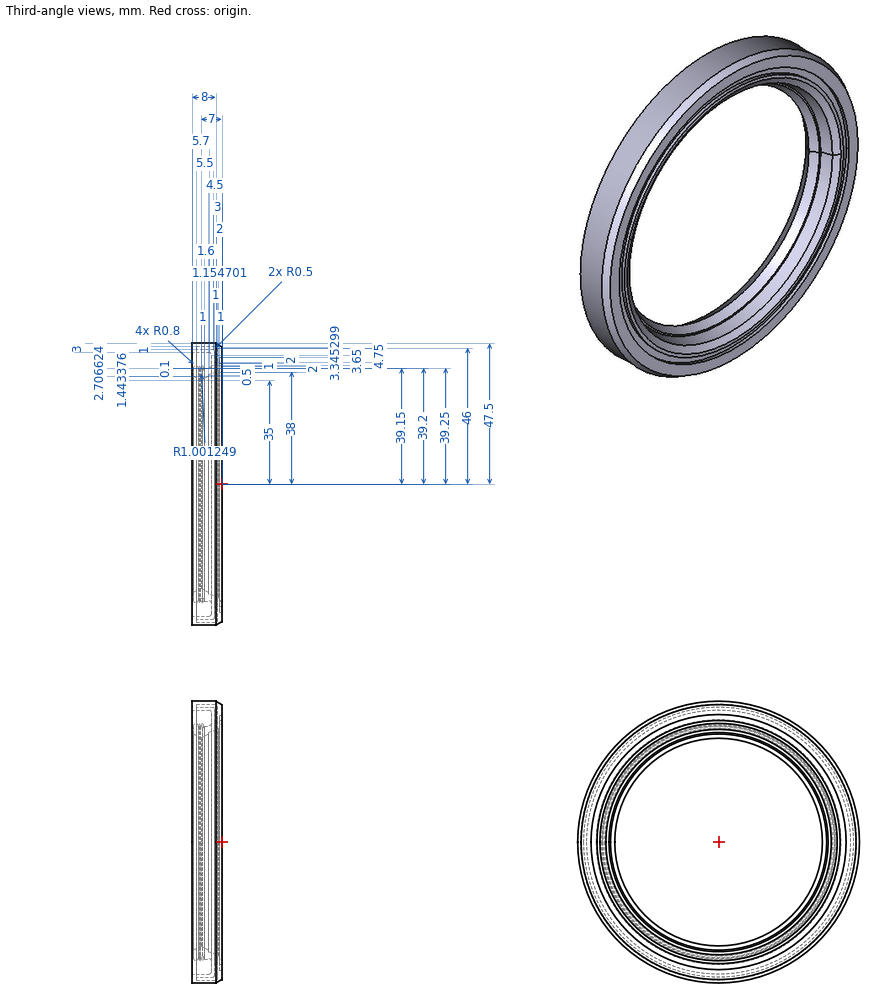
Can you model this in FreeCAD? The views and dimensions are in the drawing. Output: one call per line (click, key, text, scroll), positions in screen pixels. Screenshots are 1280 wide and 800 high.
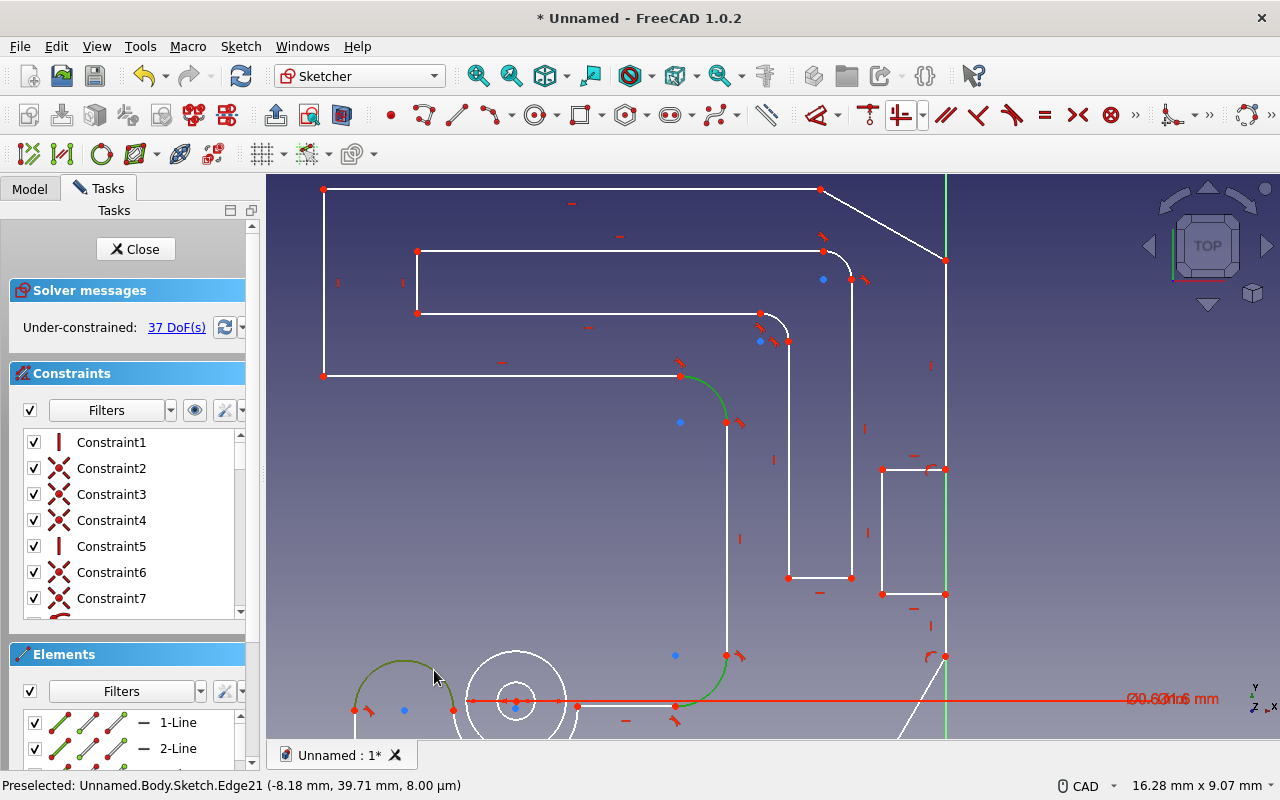
click(1045, 116)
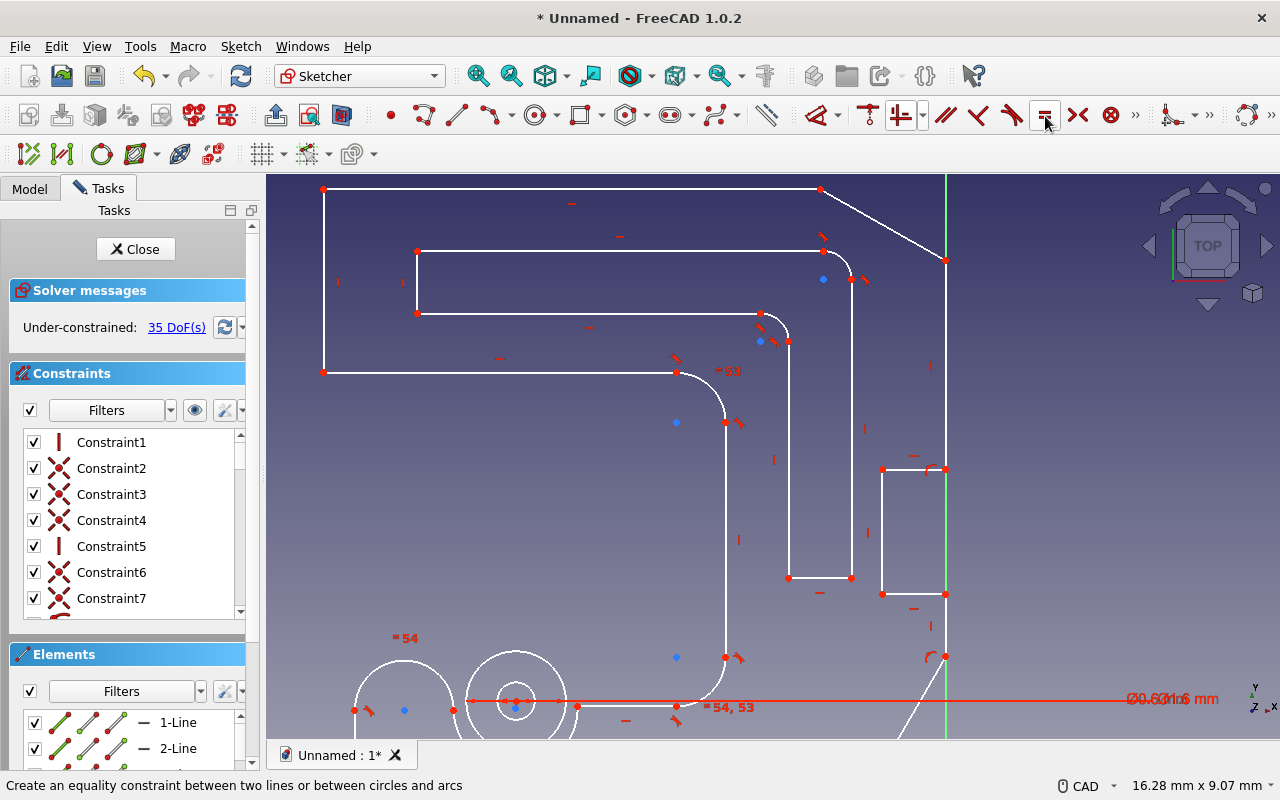
click(848, 266)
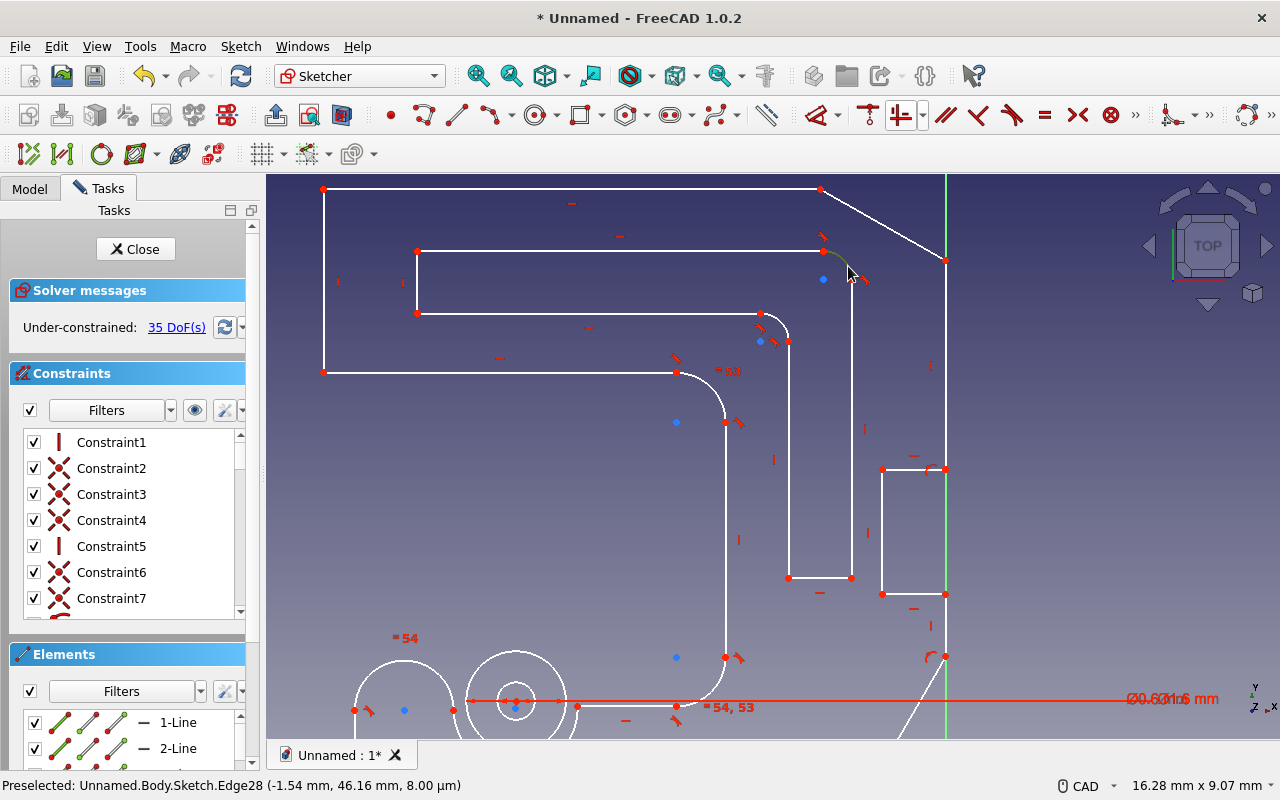
click(786, 329)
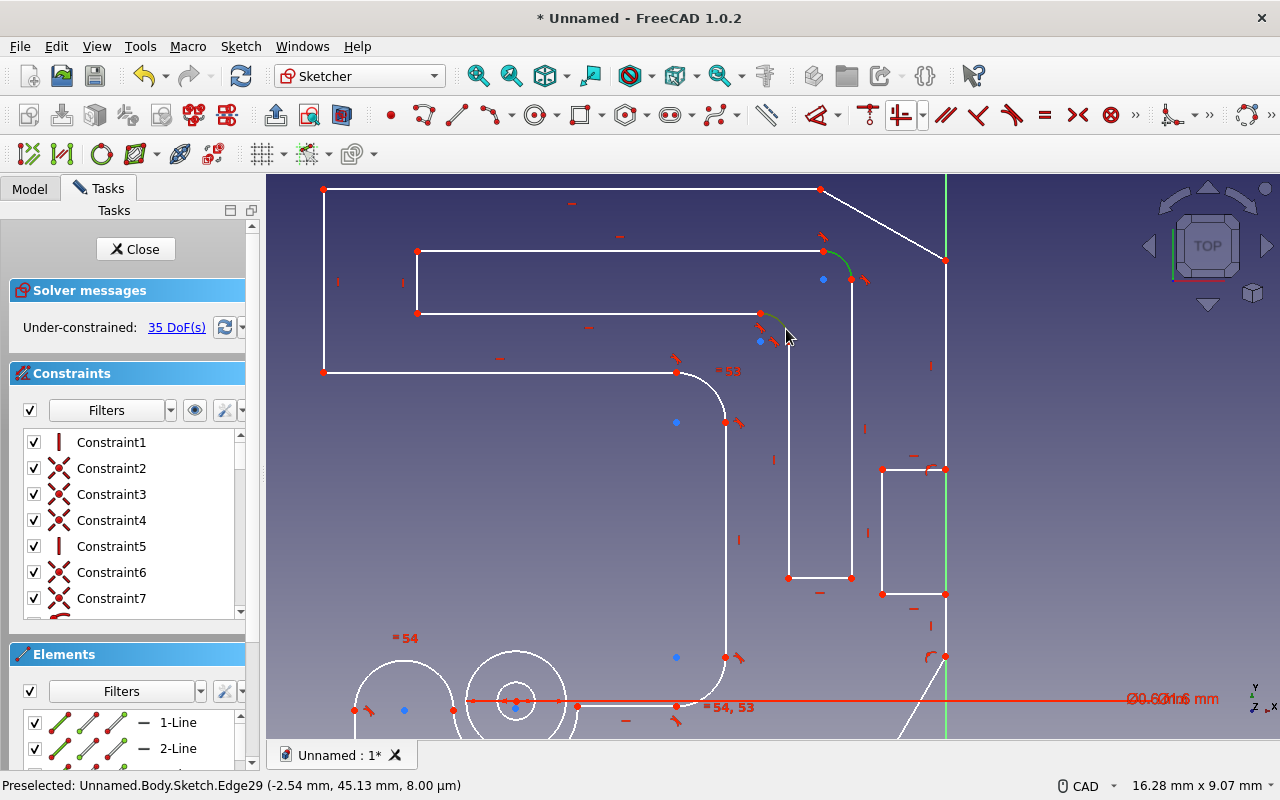
key(e)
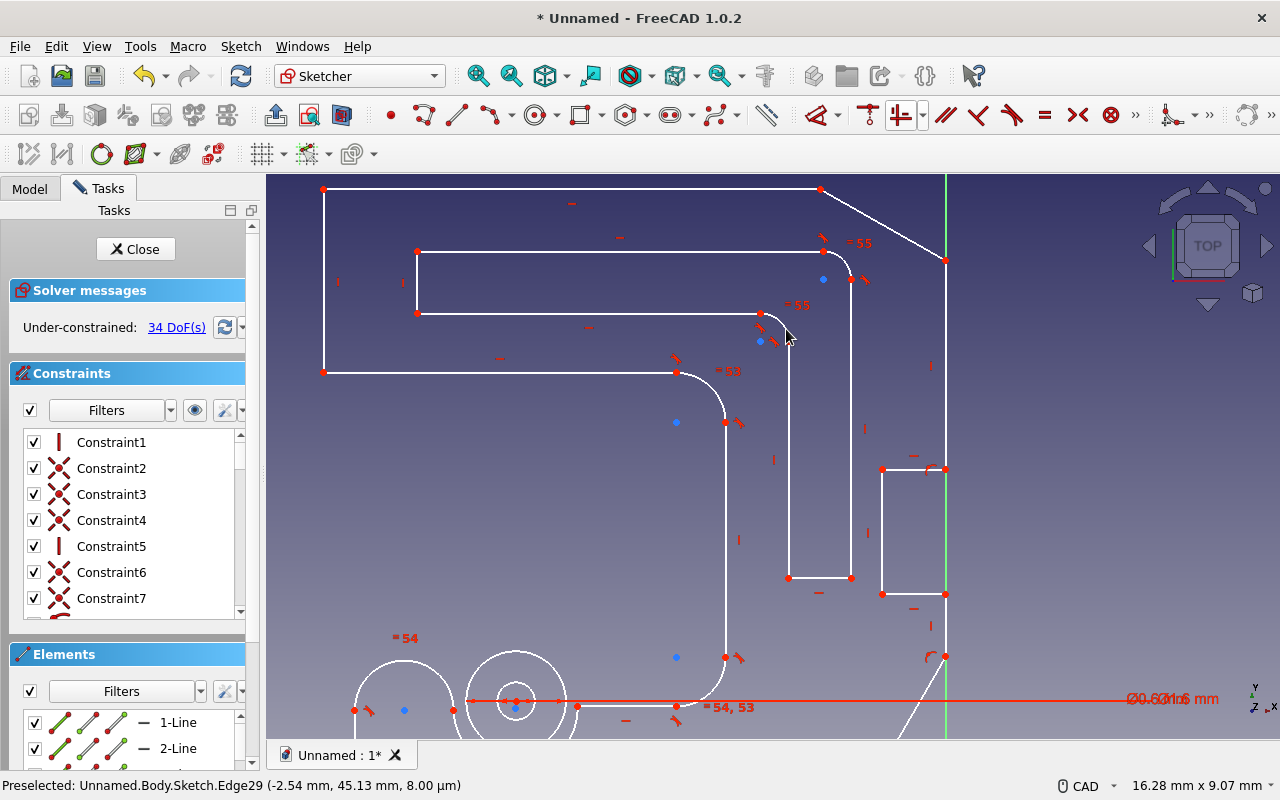
click(816, 116)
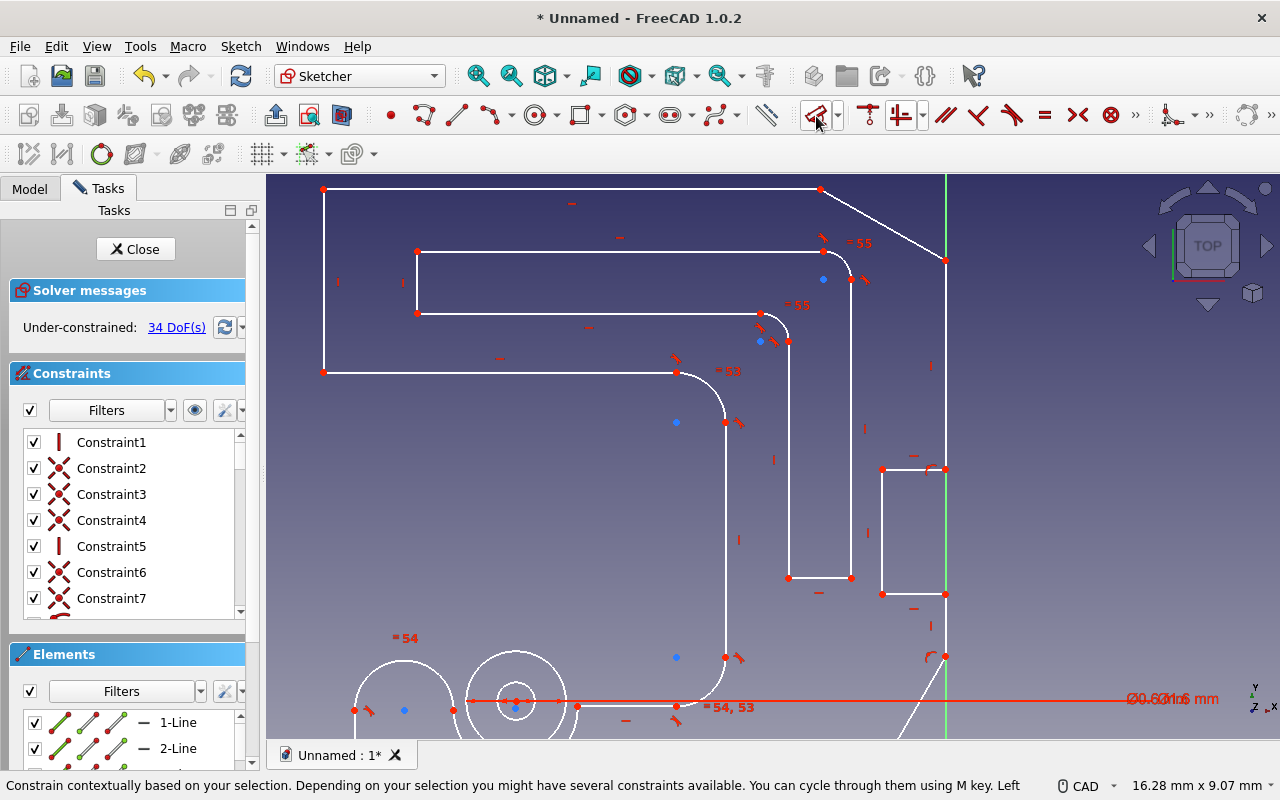
click(720, 400)
click(749, 385)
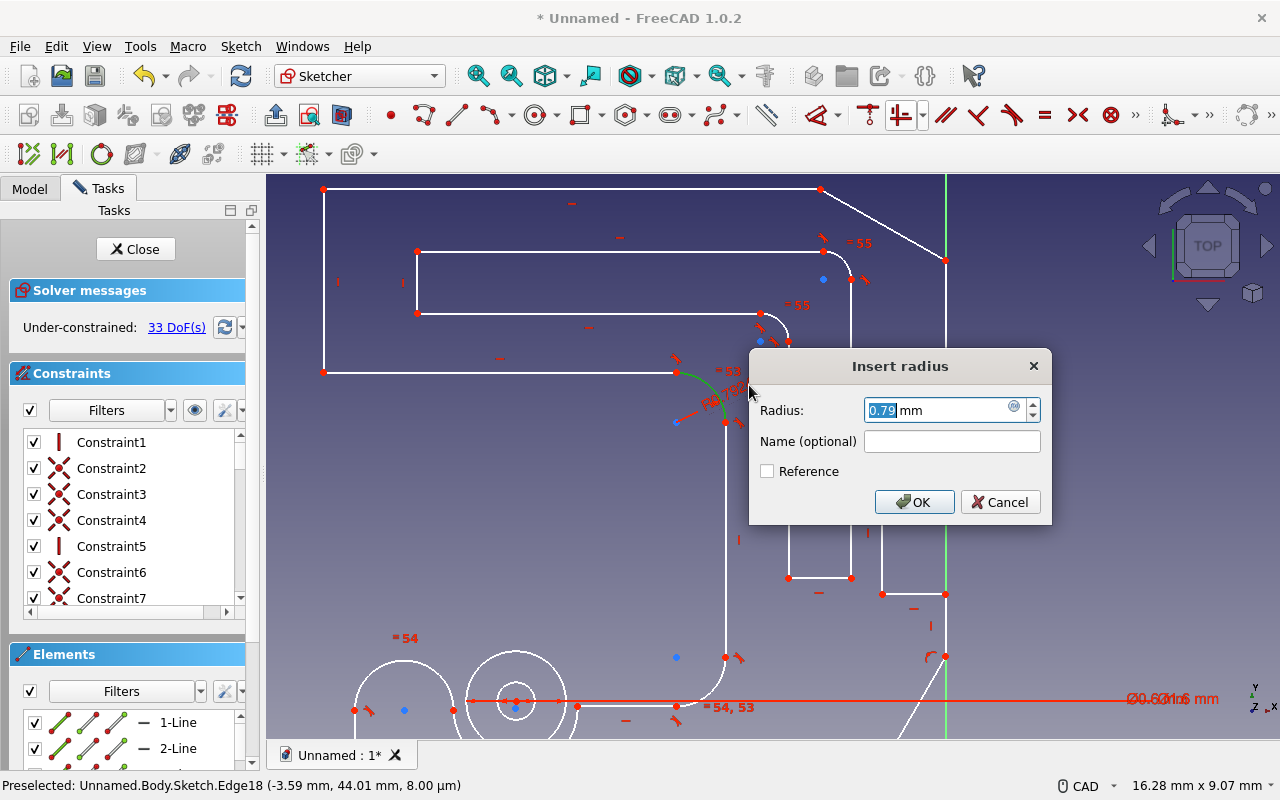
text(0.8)
key(Return)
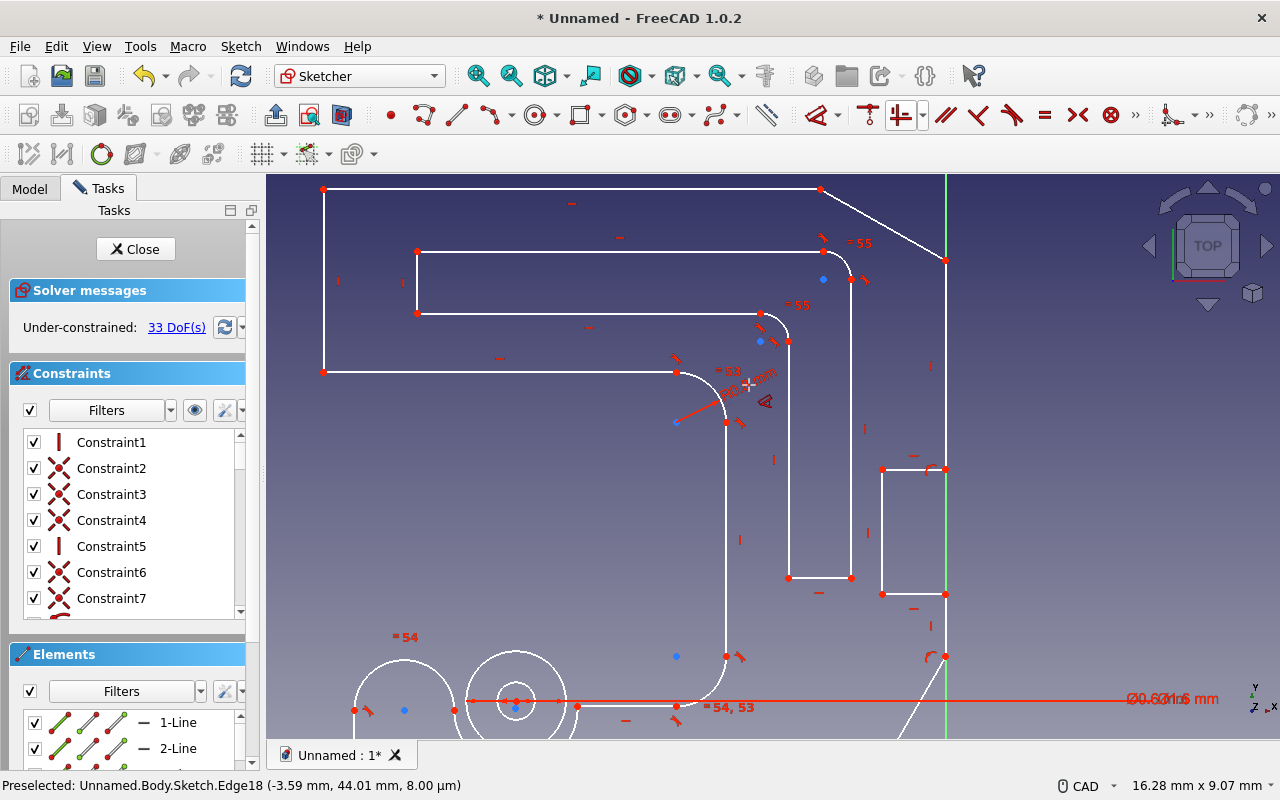
scroll(762, 359, down, 4)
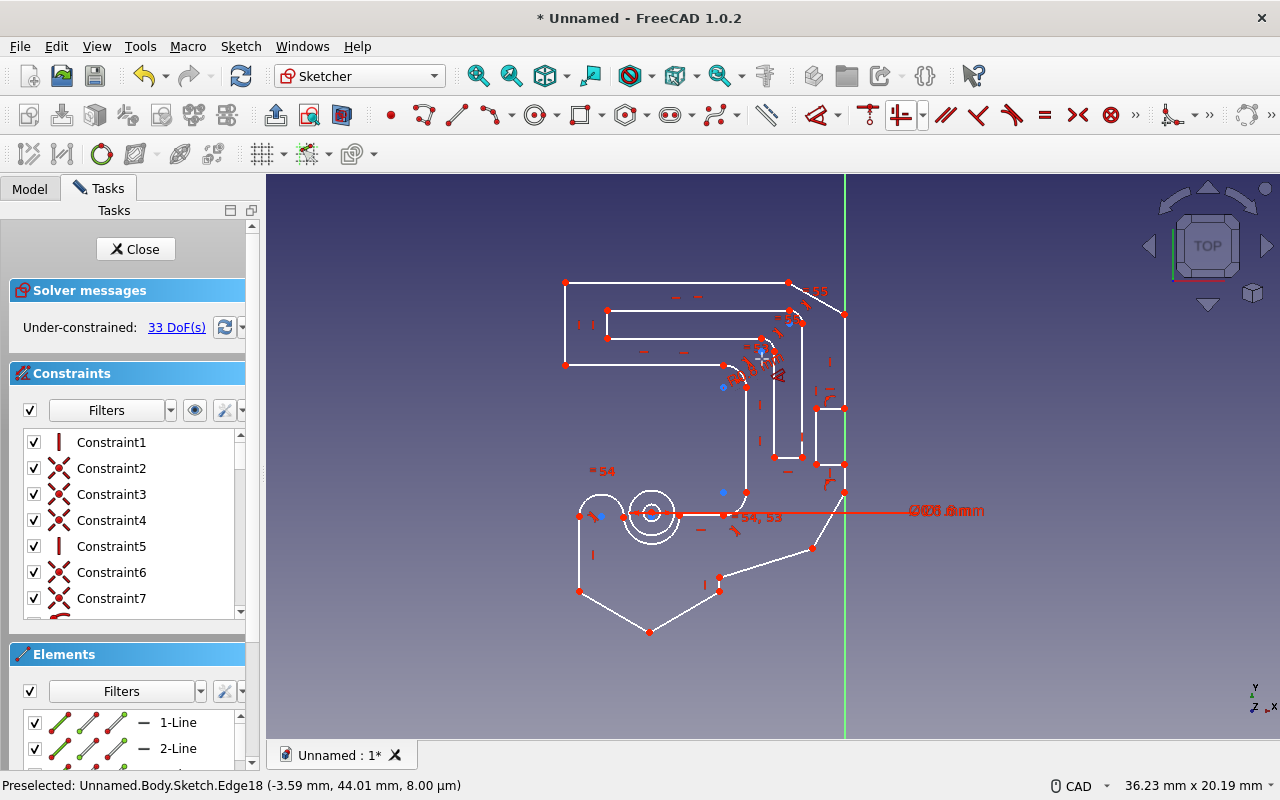
scroll(636, 539, up, 3)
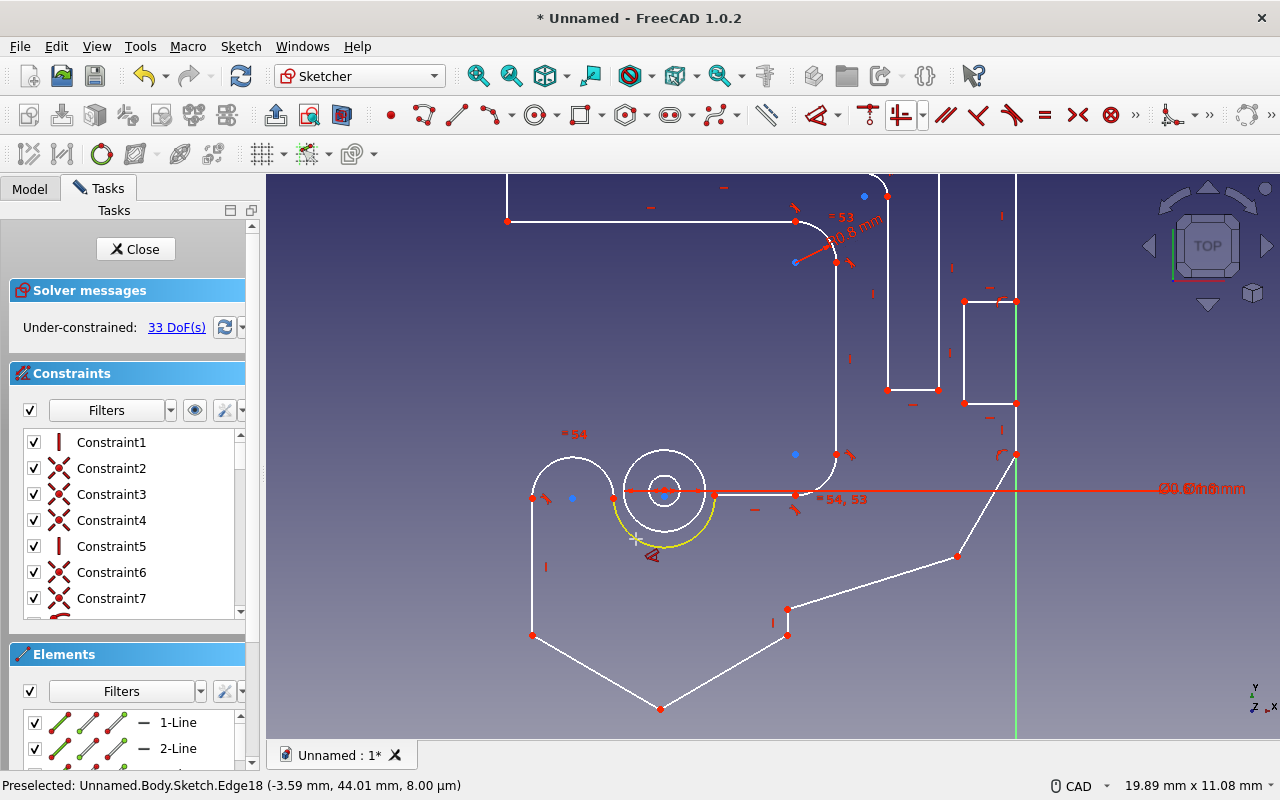
click(636, 539)
click(618, 566)